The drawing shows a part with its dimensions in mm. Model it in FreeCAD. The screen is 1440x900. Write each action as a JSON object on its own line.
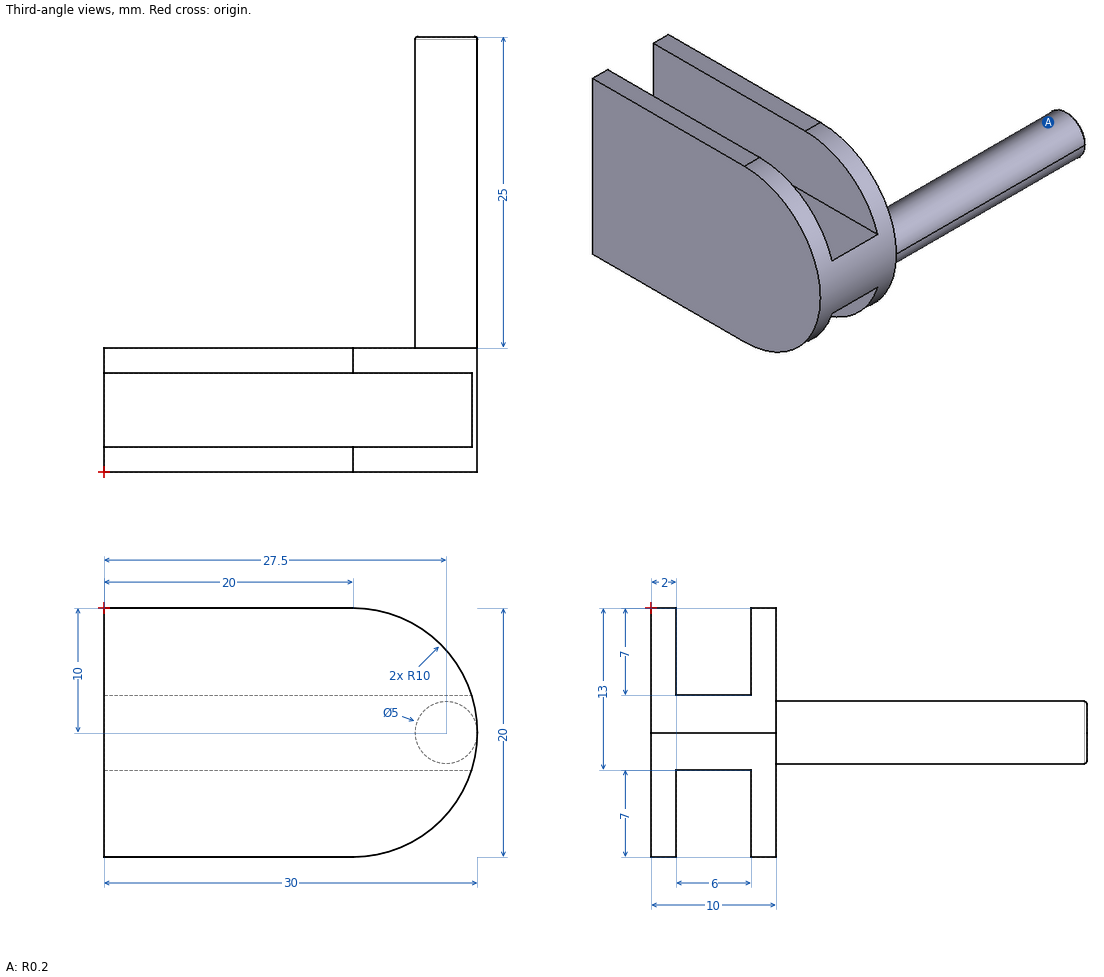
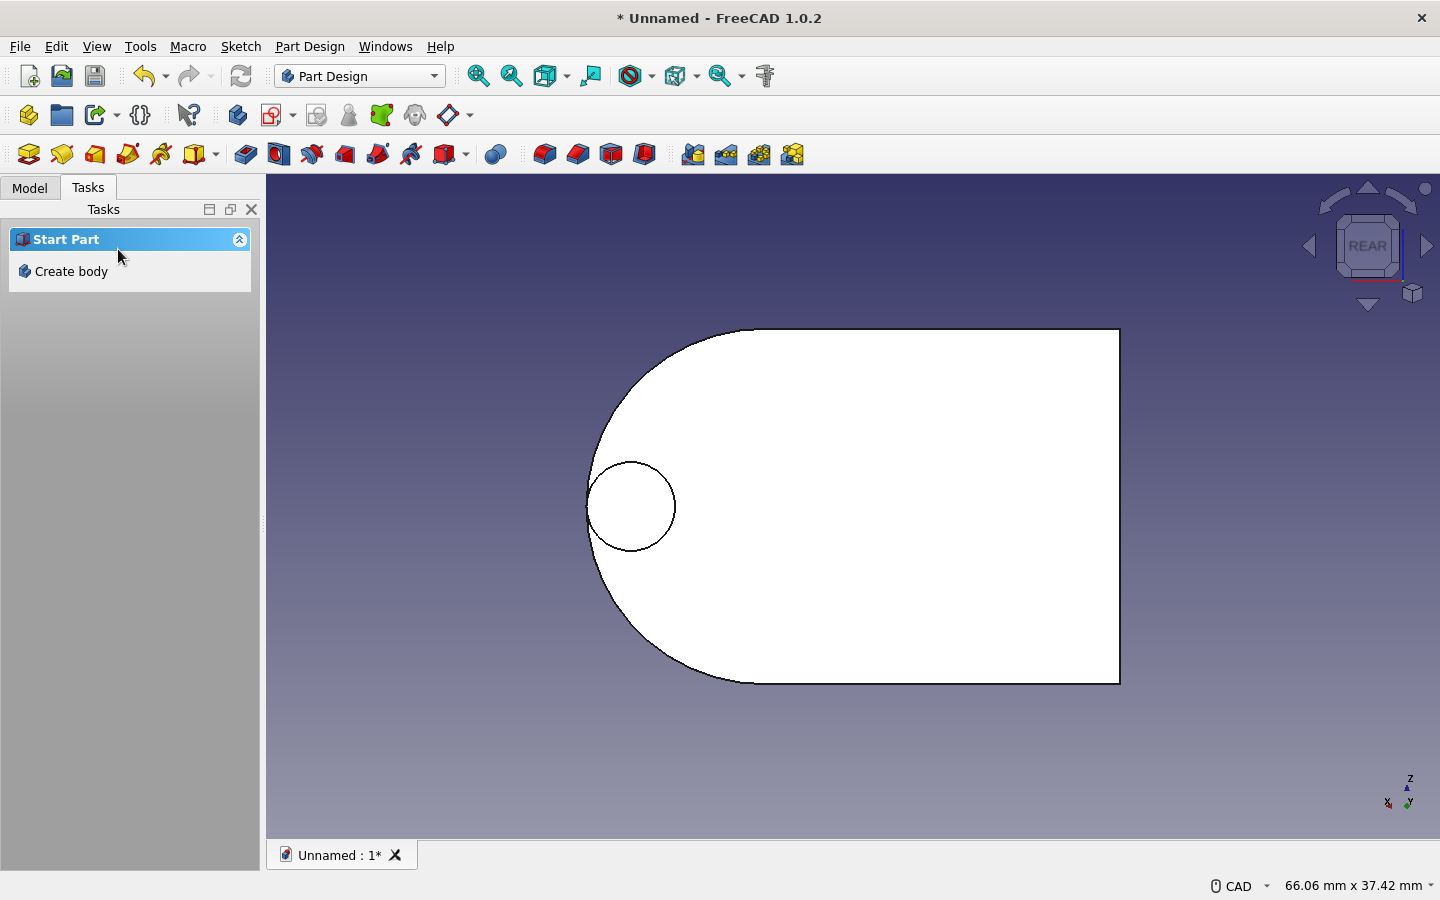
{"action": "left_click", "coordinate": [675, 506]}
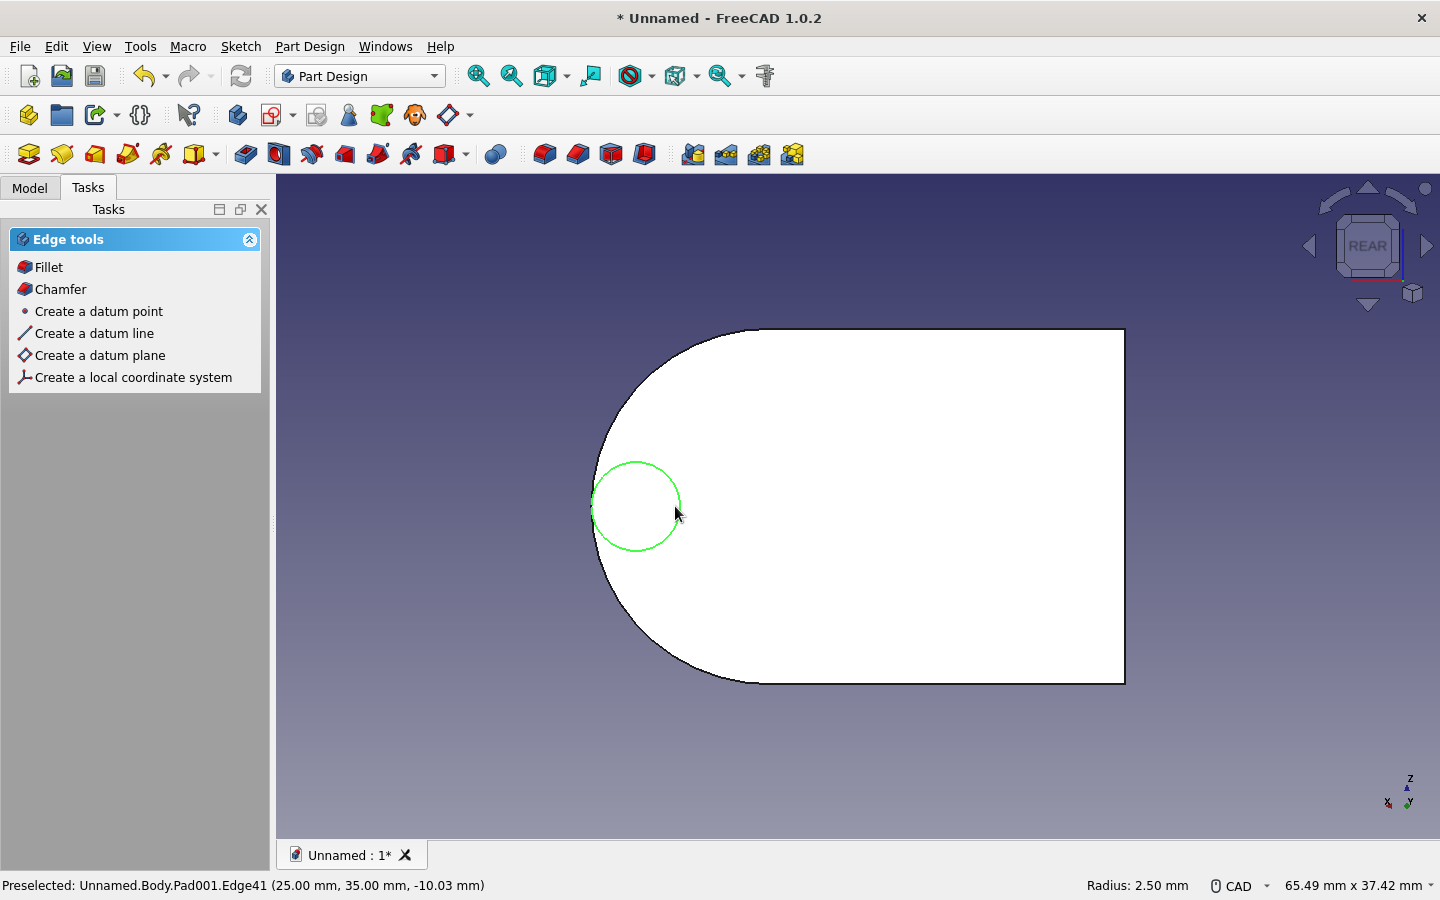
{"action": "left_click", "coordinate": [545, 154]}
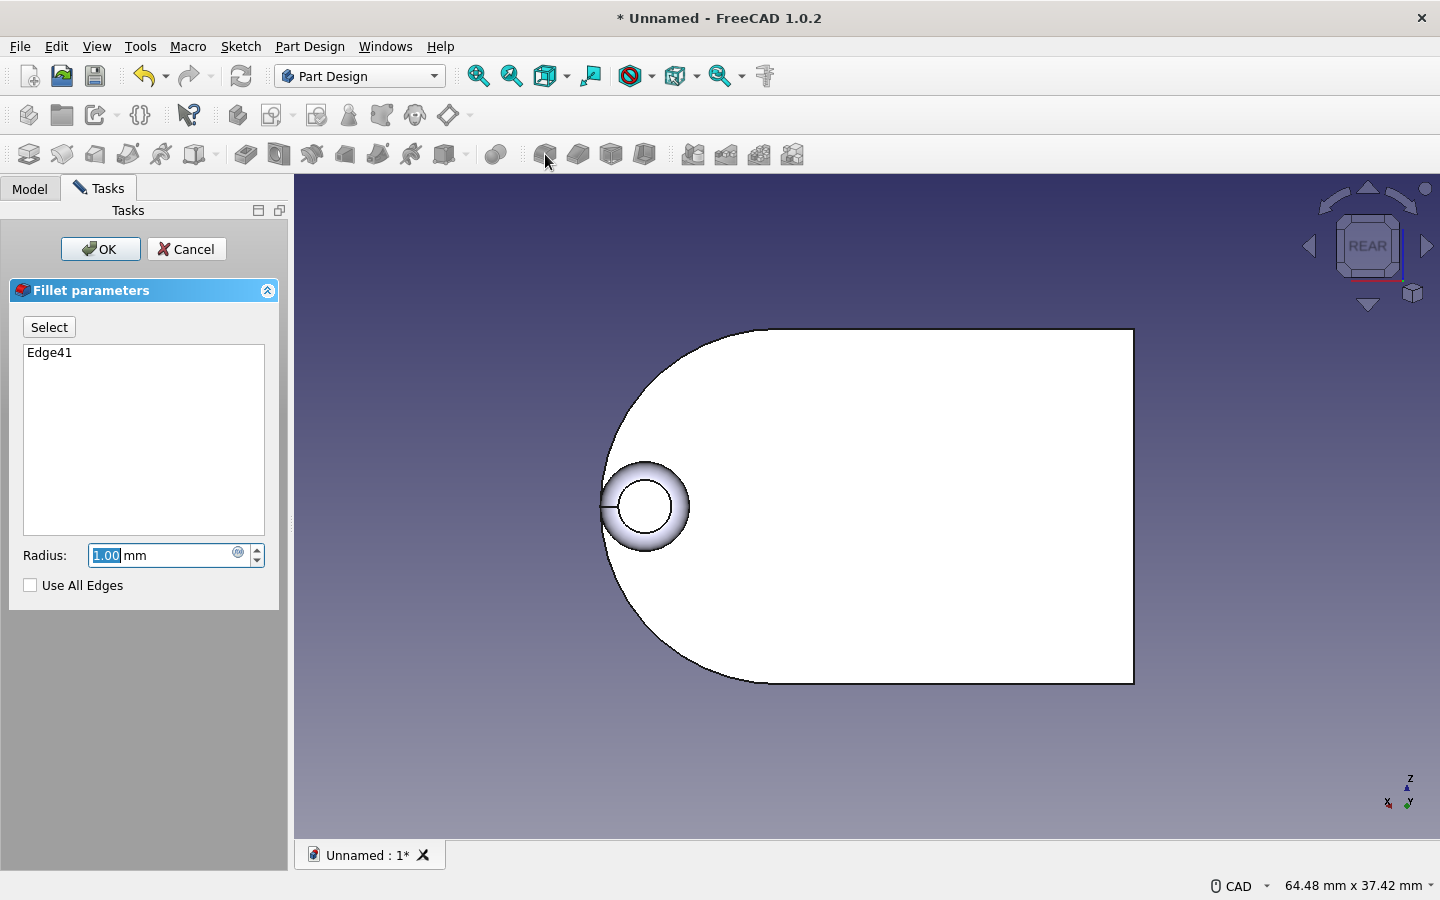
{"action": "type", "text": "0.2"}
{"action": "key", "text": "Tab"}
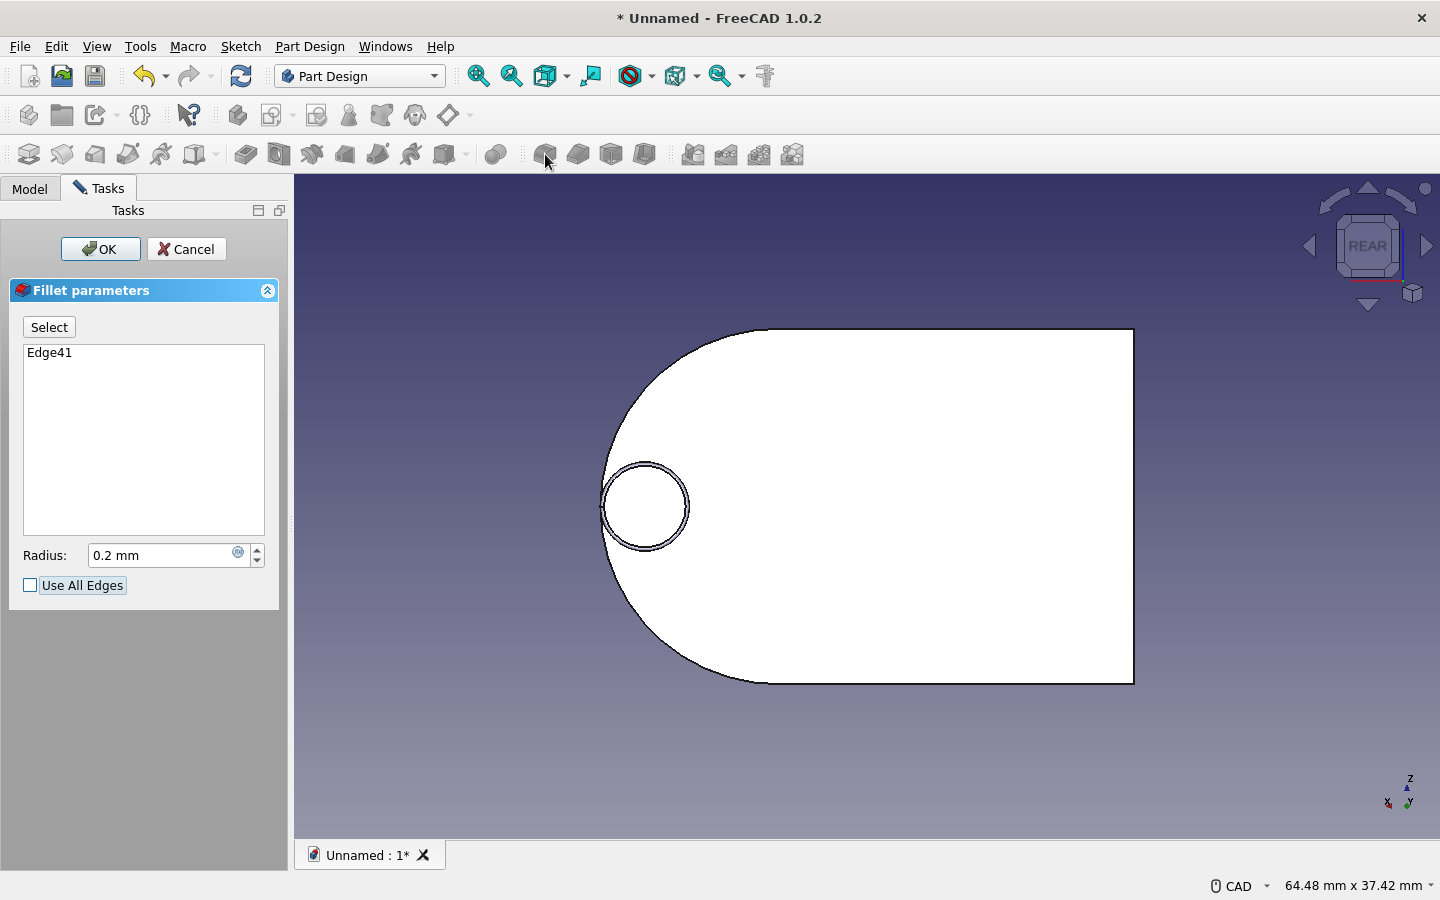
{"action": "left_click", "coordinate": [101, 249]}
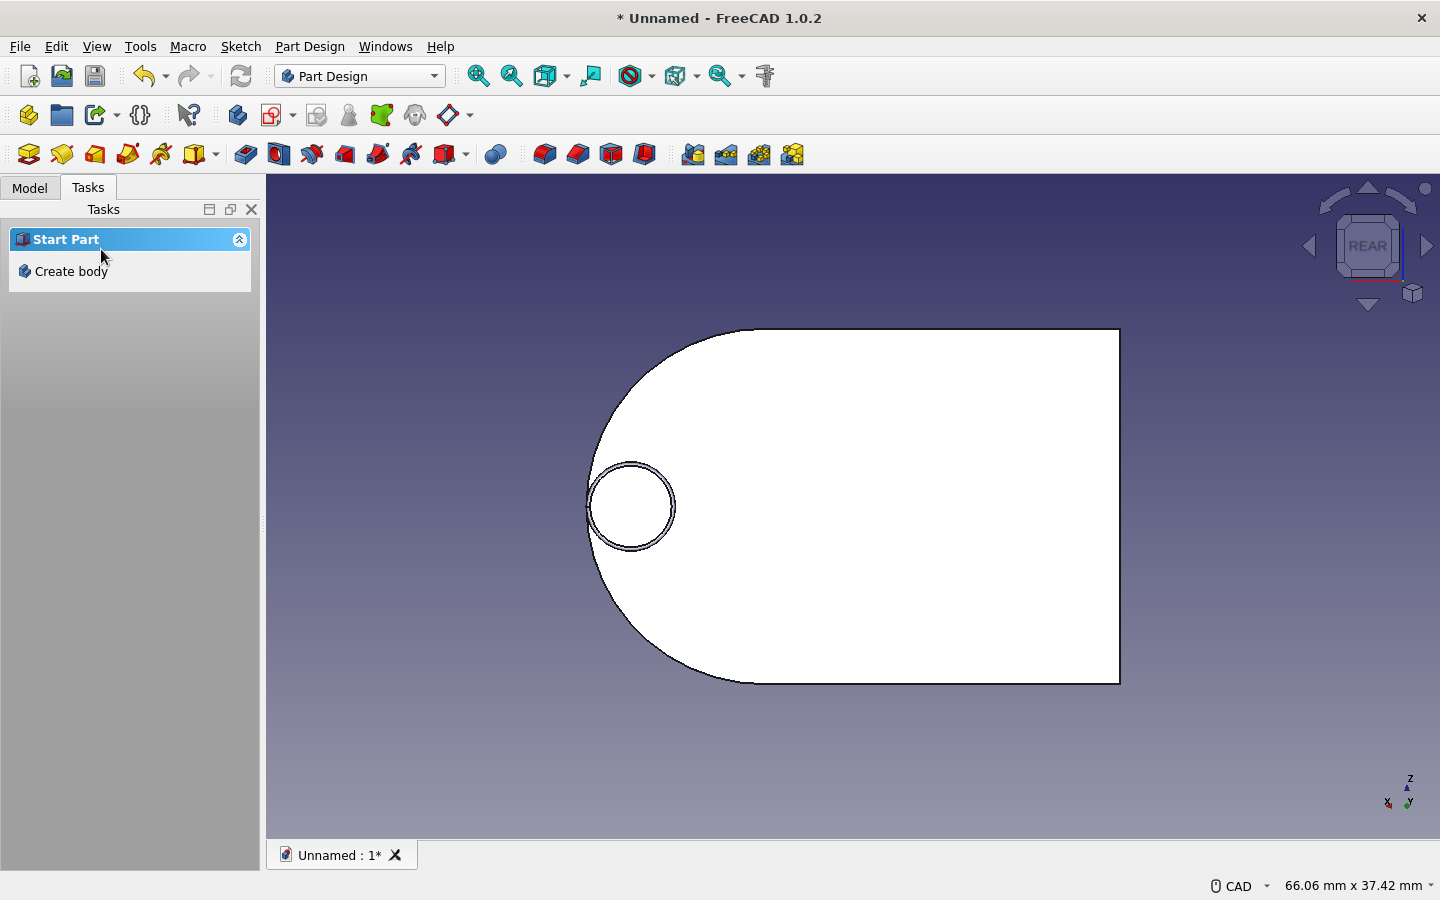
{"action": "key", "text": "0"}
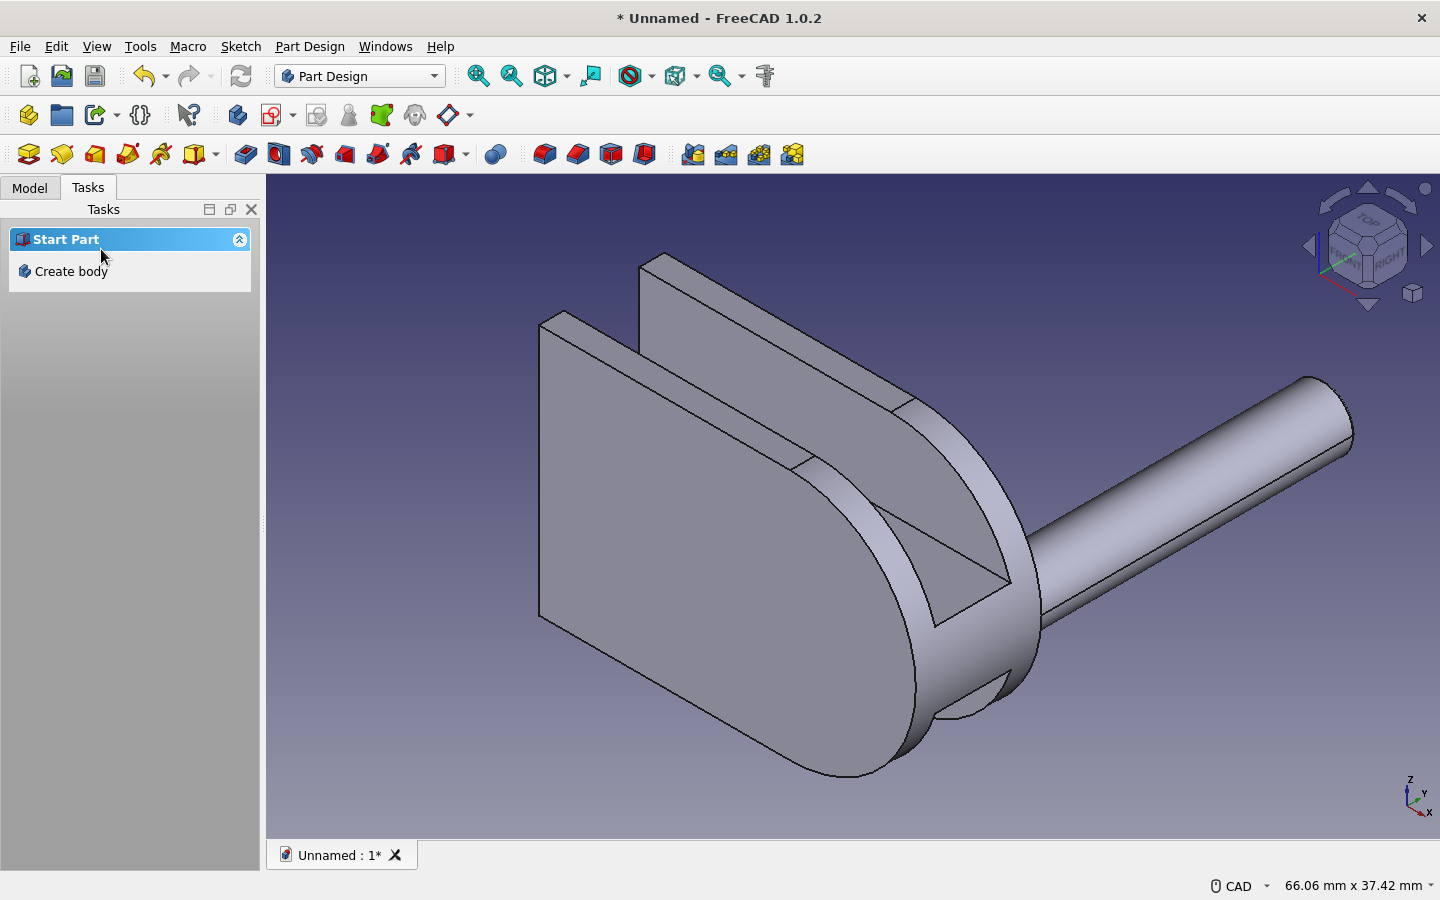
{"action": "left_click", "coordinate": [479, 76]}